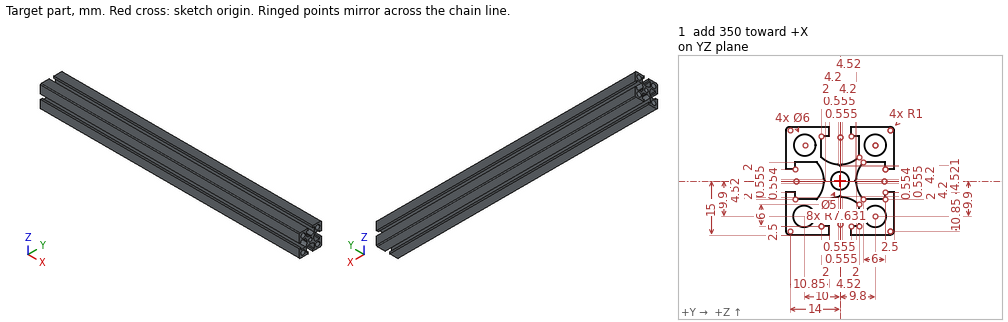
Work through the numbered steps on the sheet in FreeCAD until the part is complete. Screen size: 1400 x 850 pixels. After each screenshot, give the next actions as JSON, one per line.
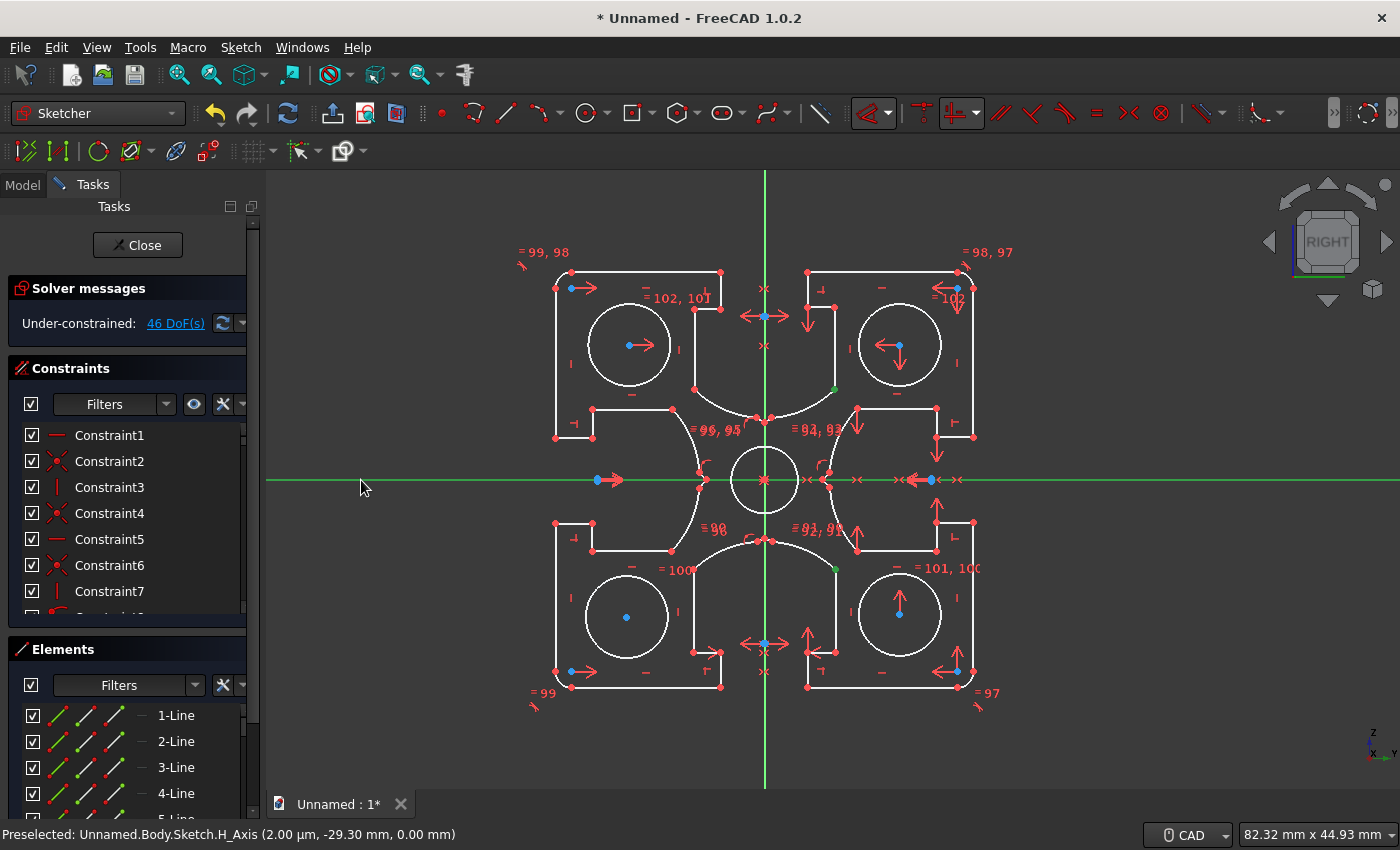
{"action": "left_click", "coordinate": [1130, 114]}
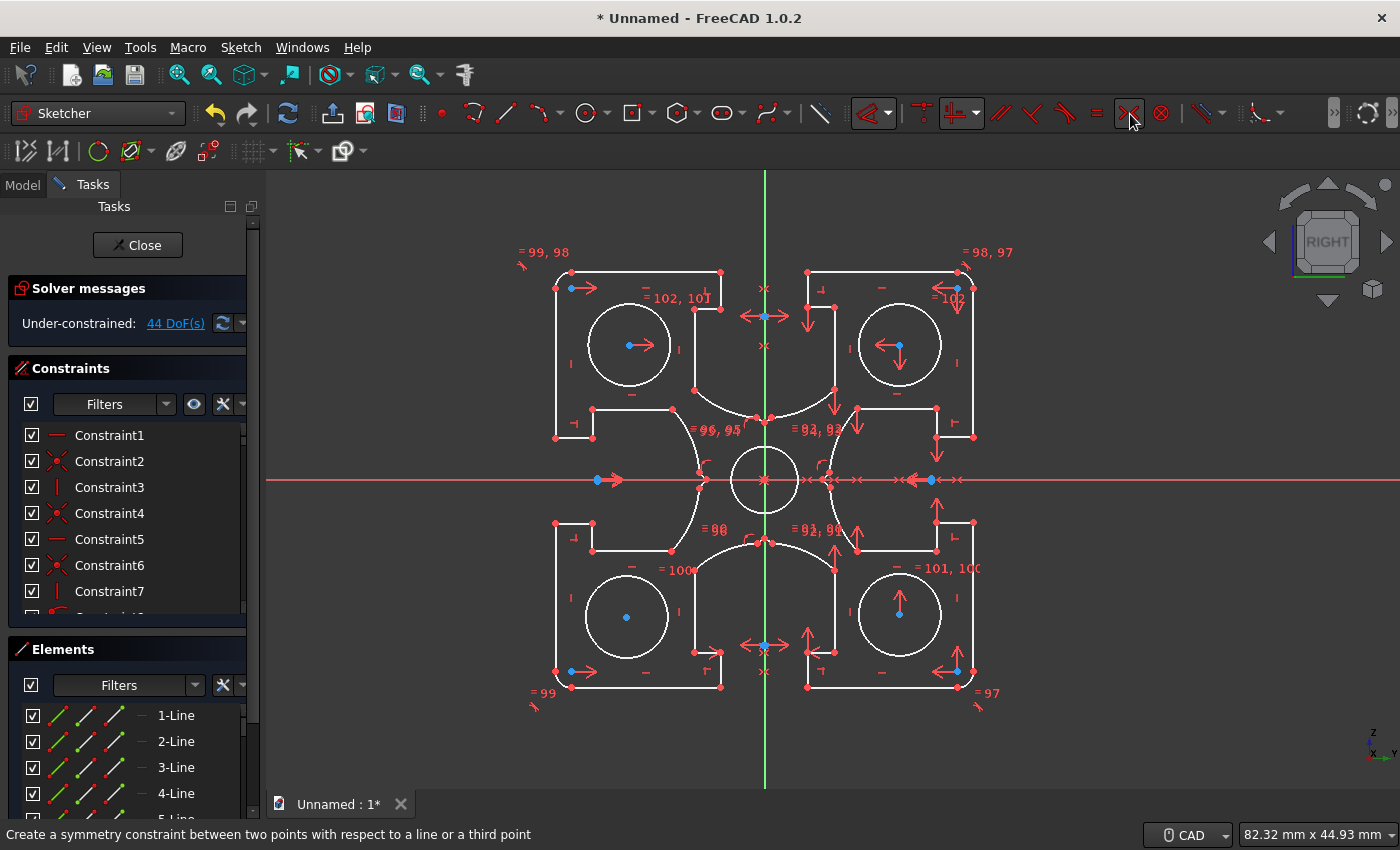
{"action": "left_click", "coordinate": [695, 653]}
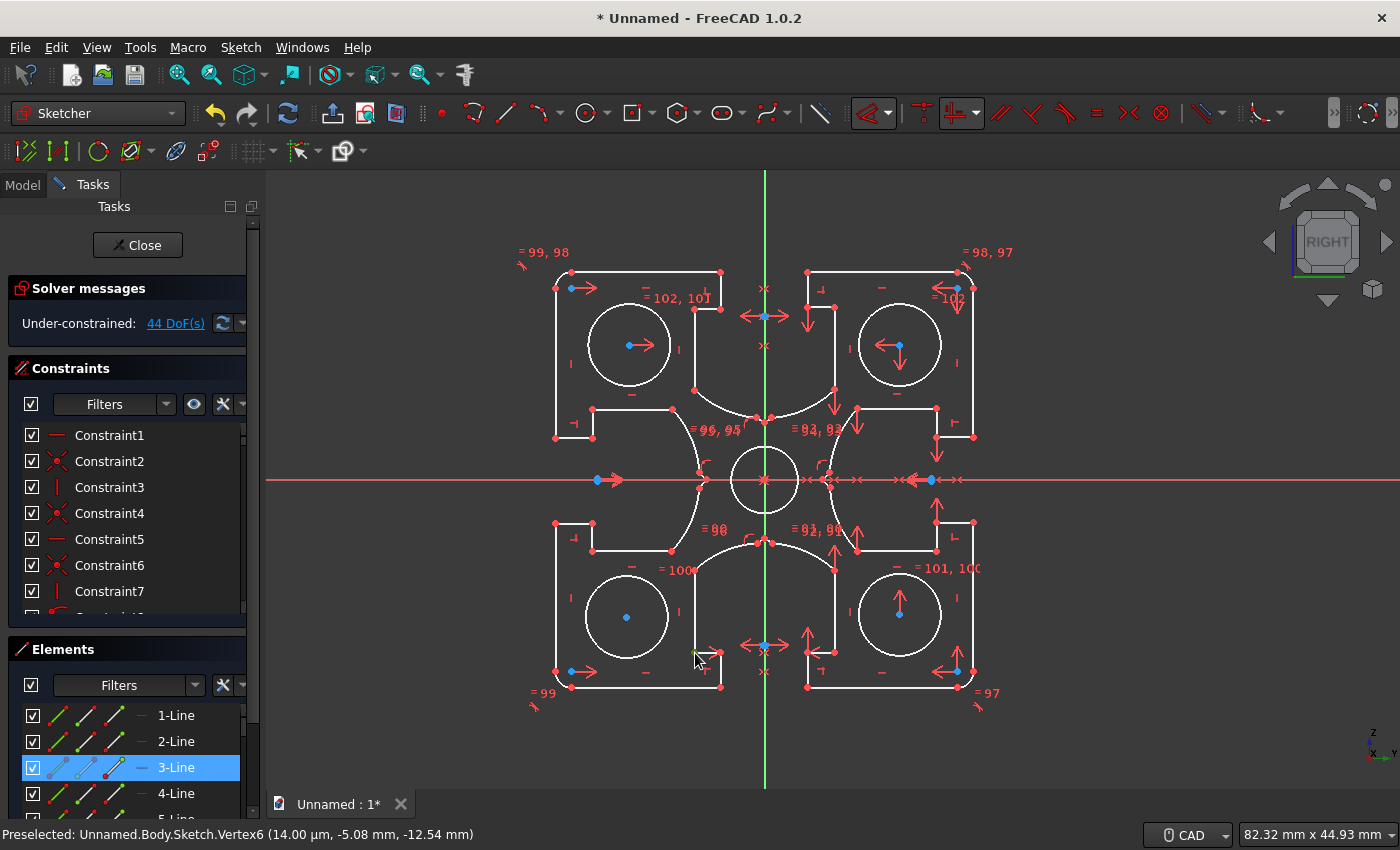
{"action": "left_click", "coordinate": [695, 309]}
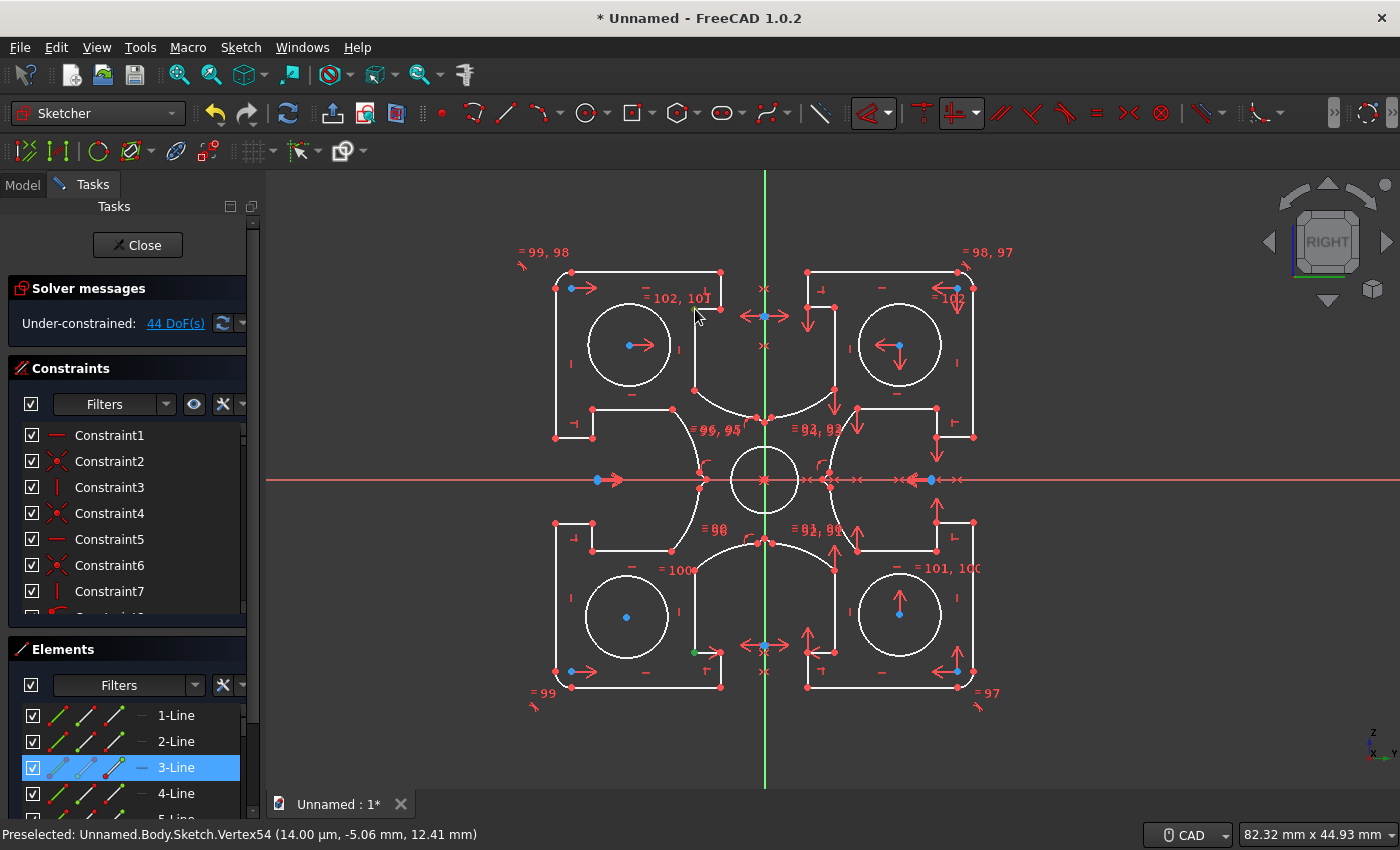
{"action": "left_click", "coordinate": [361, 480]}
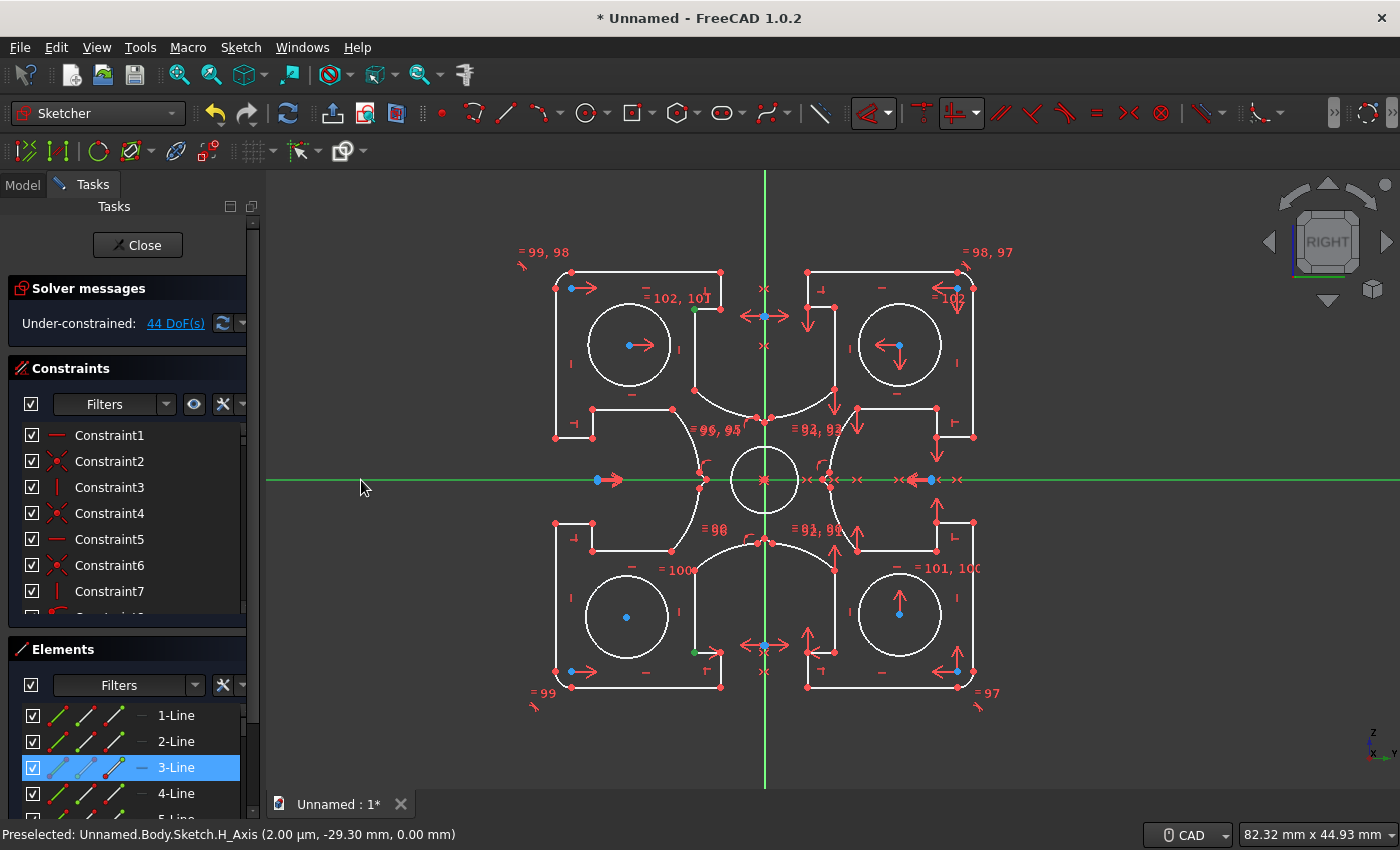
{"action": "left_click", "coordinate": [1130, 114]}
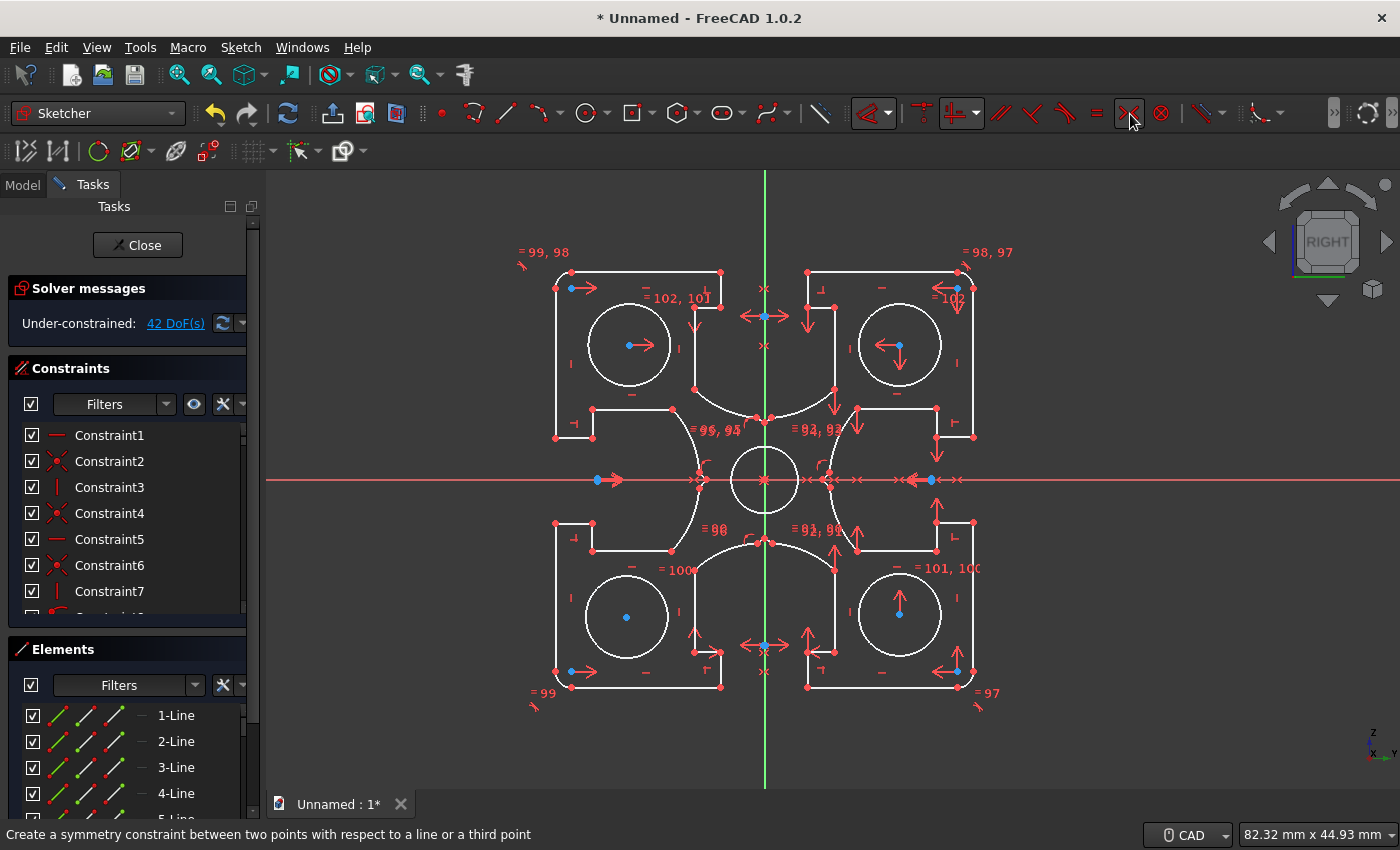
{"action": "left_click", "coordinate": [937, 437]}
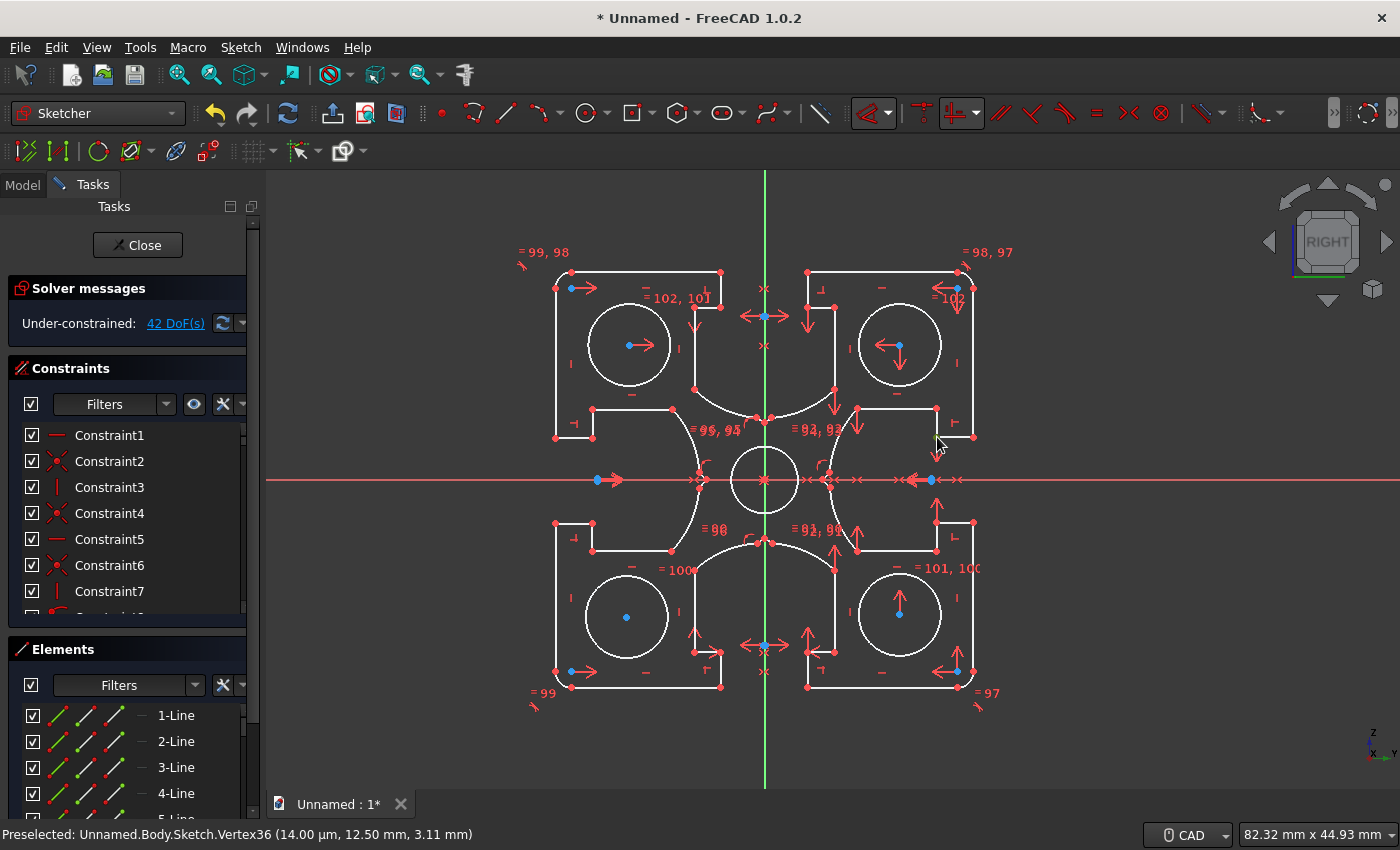
{"action": "left_click", "coordinate": [593, 438]}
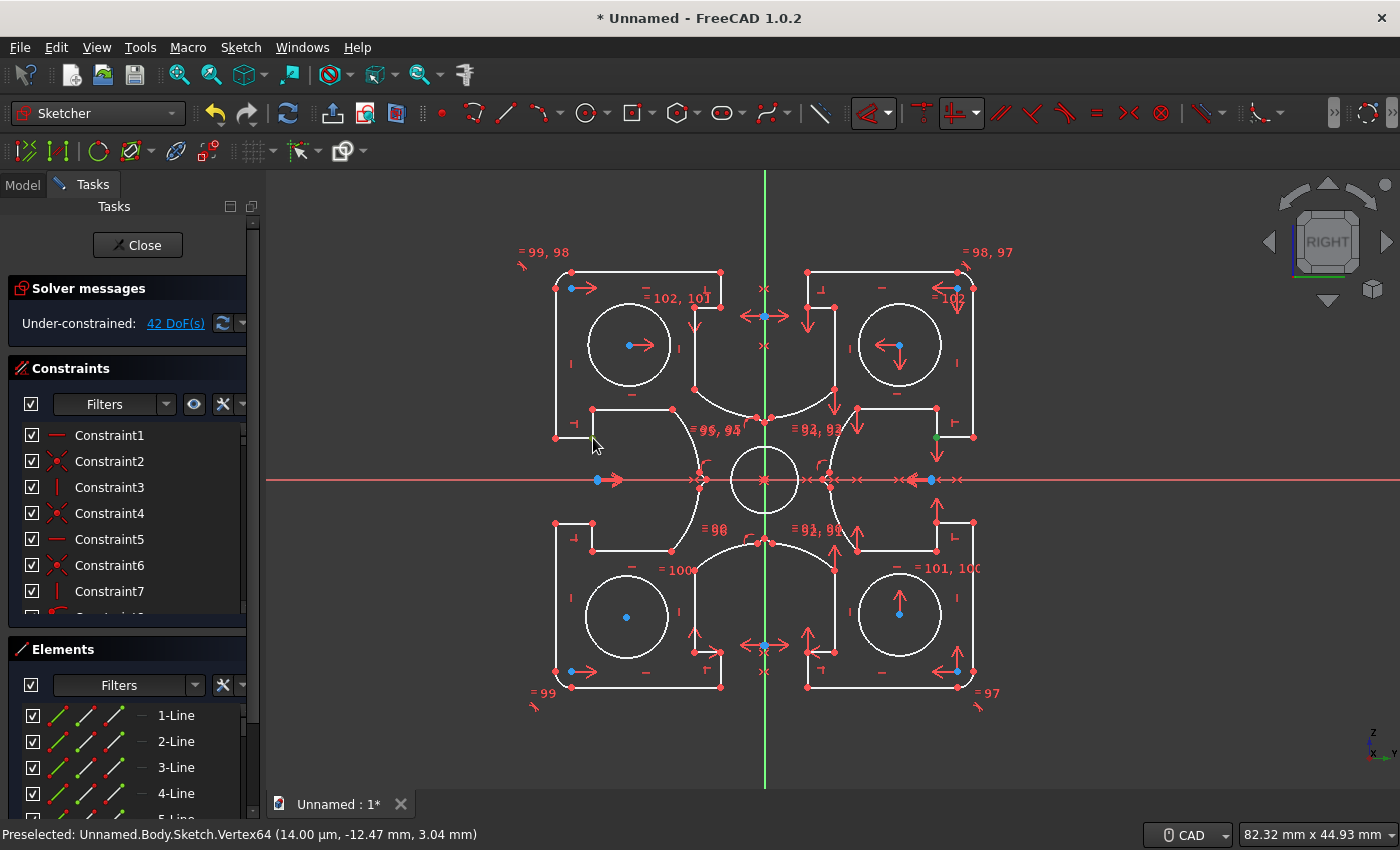
{"action": "left_click", "coordinate": [765, 721]}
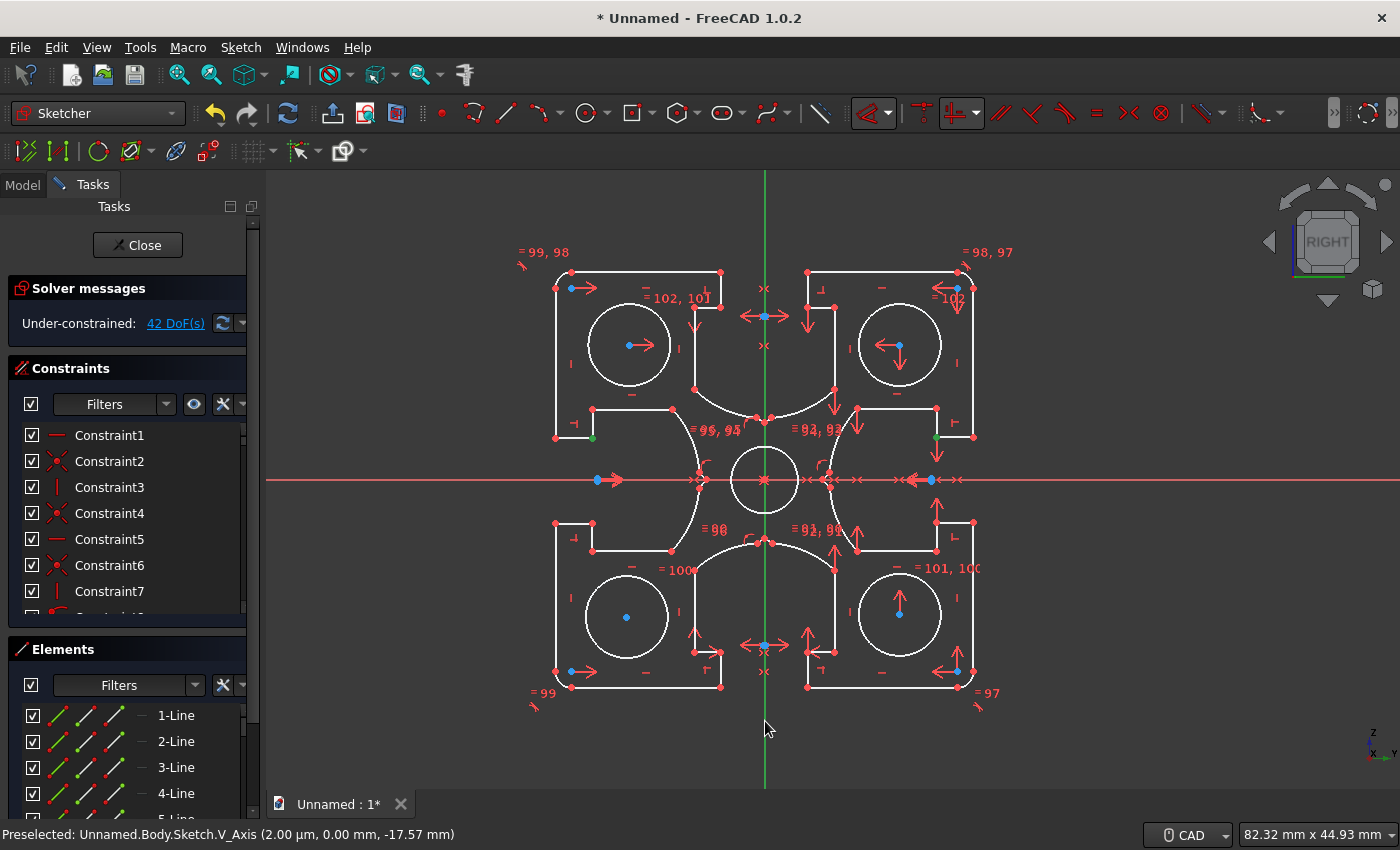
{"action": "left_click", "coordinate": [1130, 114]}